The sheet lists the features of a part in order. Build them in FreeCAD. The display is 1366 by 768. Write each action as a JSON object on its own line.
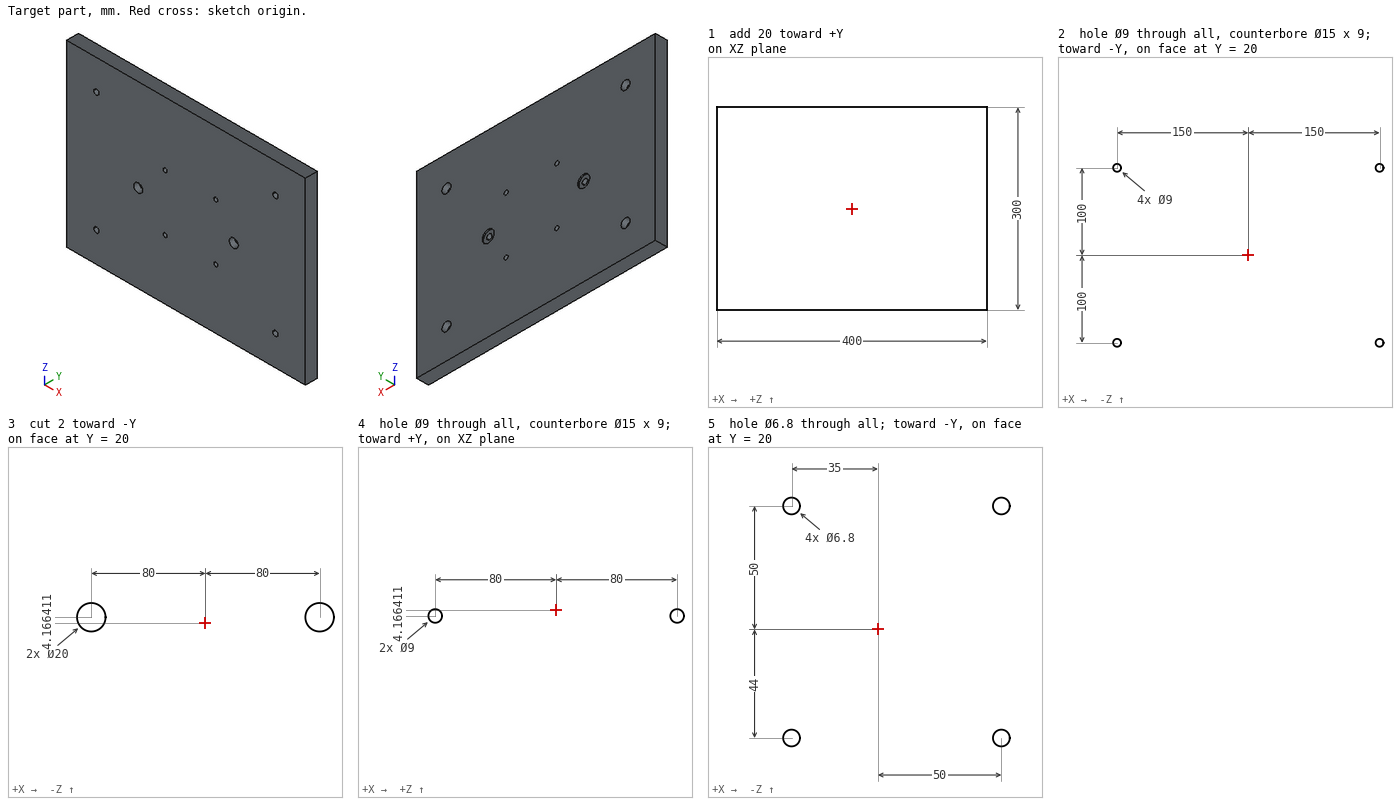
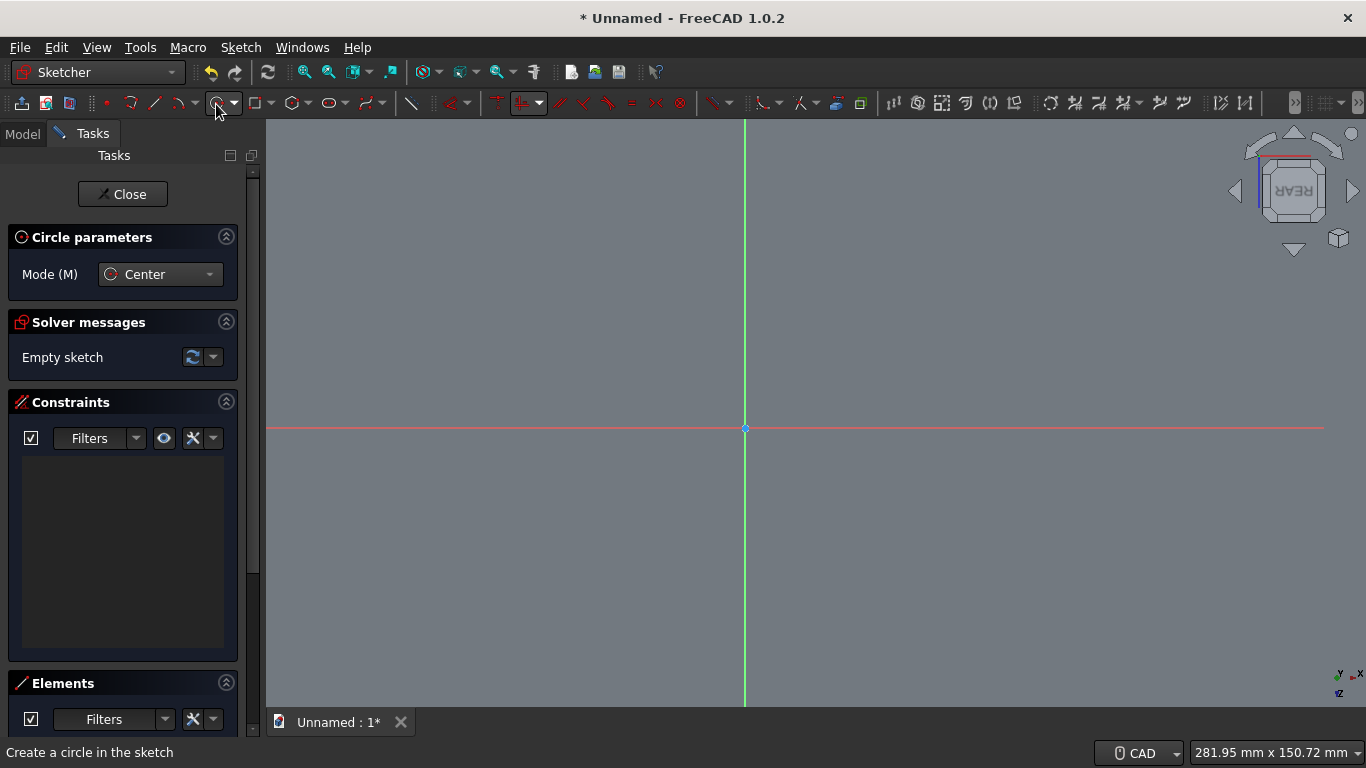
{"action": "left_click", "coordinate": [433, 412]}
{"action": "left_click", "coordinate": [461, 384]}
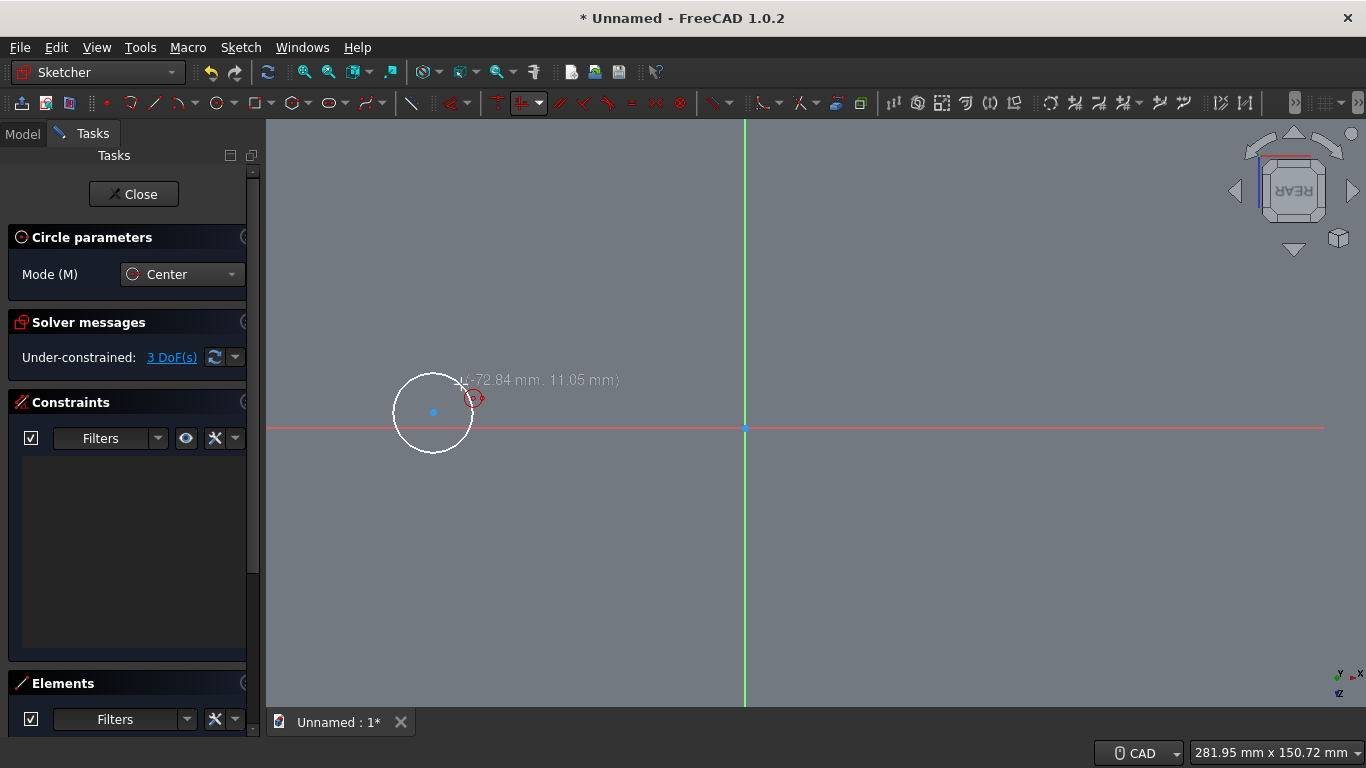
{"action": "left_click", "coordinate": [1057, 412]}
{"action": "left_click", "coordinate": [1085, 384]}
{"action": "key", "text": "Escape"}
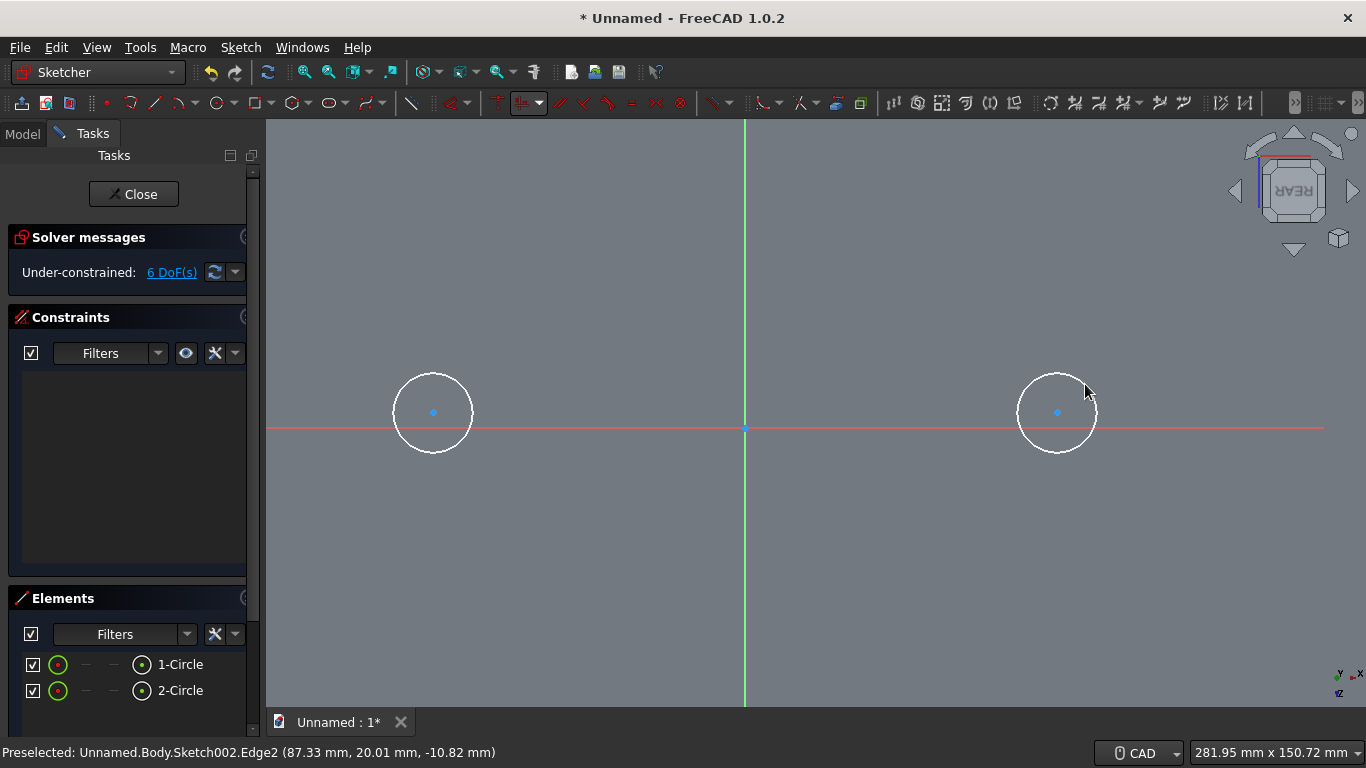
{"action": "left_click", "coordinate": [461, 385]}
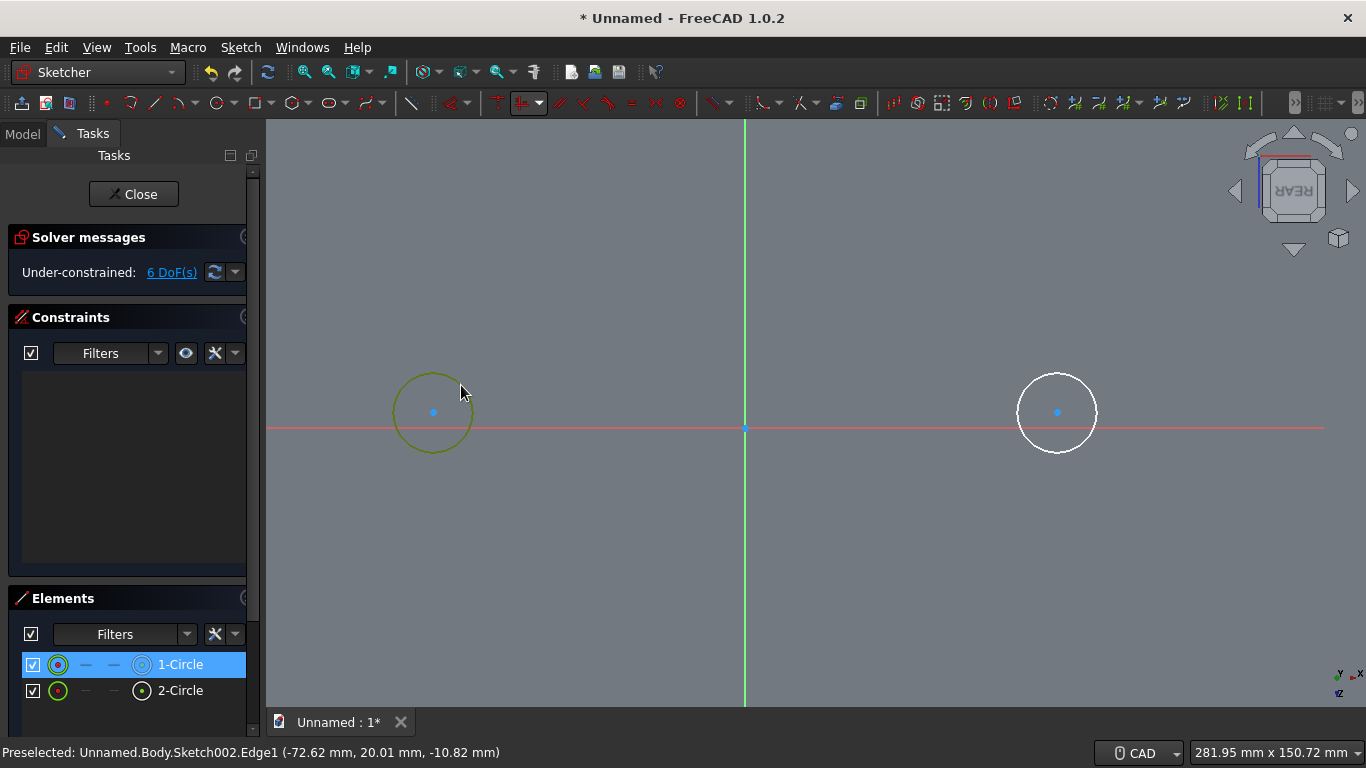
{"action": "left_click", "coordinate": [1085, 385]}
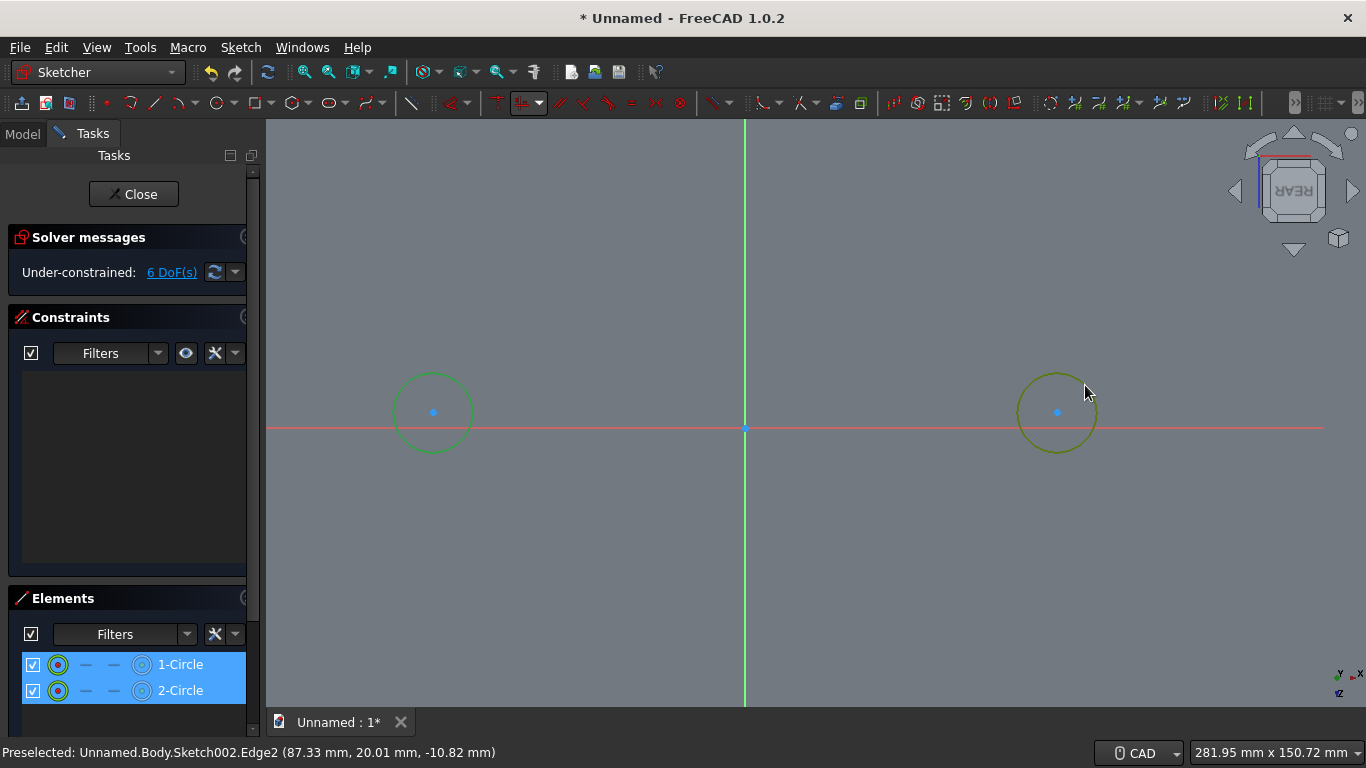
{"action": "left_click", "coordinate": [632, 104]}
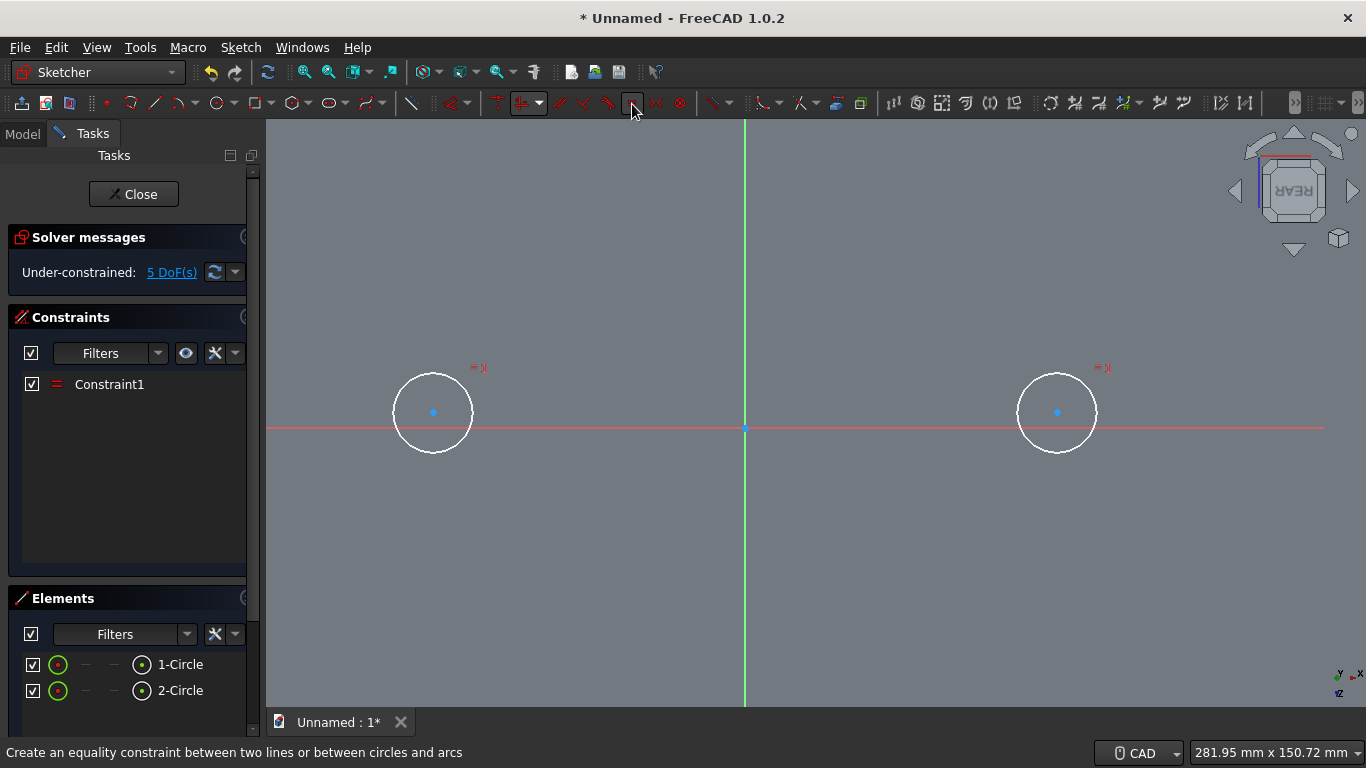
{"action": "left_click", "coordinate": [433, 413]}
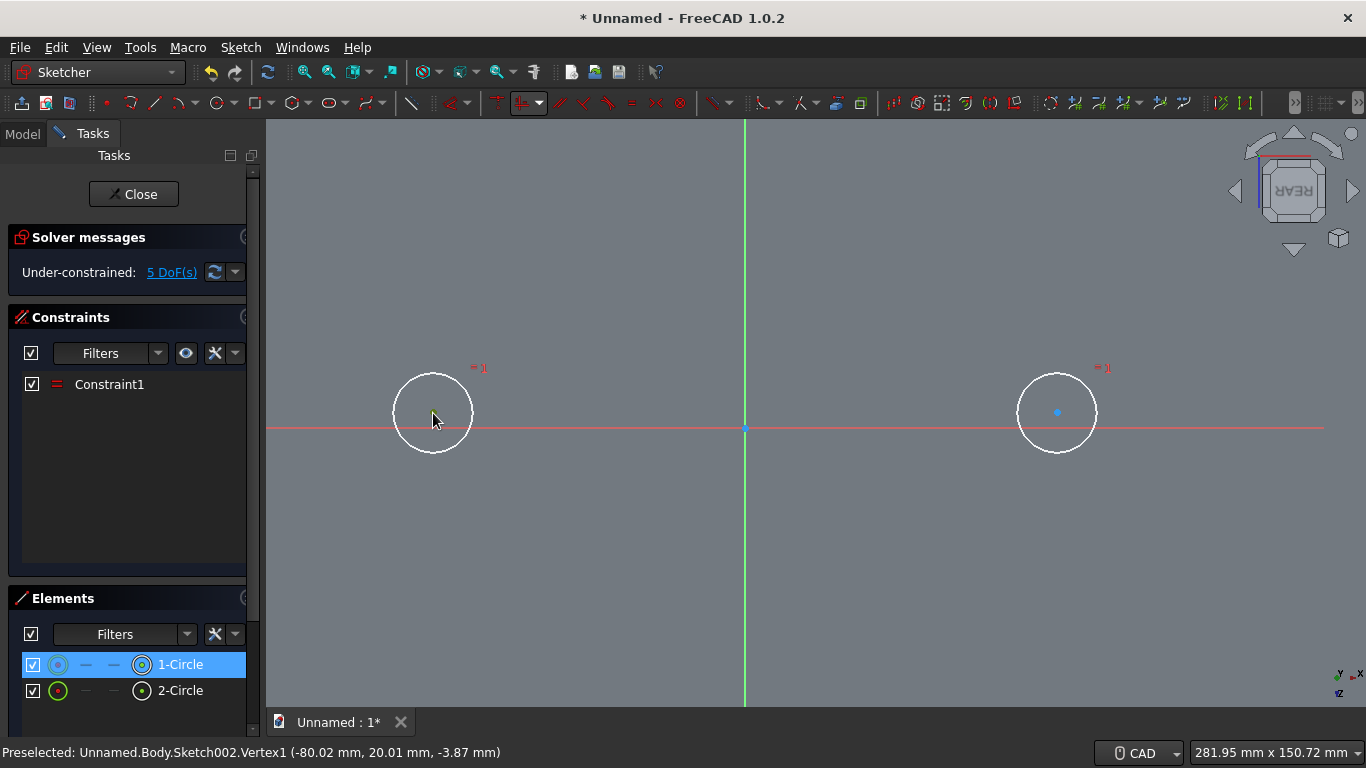
{"action": "left_click", "coordinate": [1057, 413]}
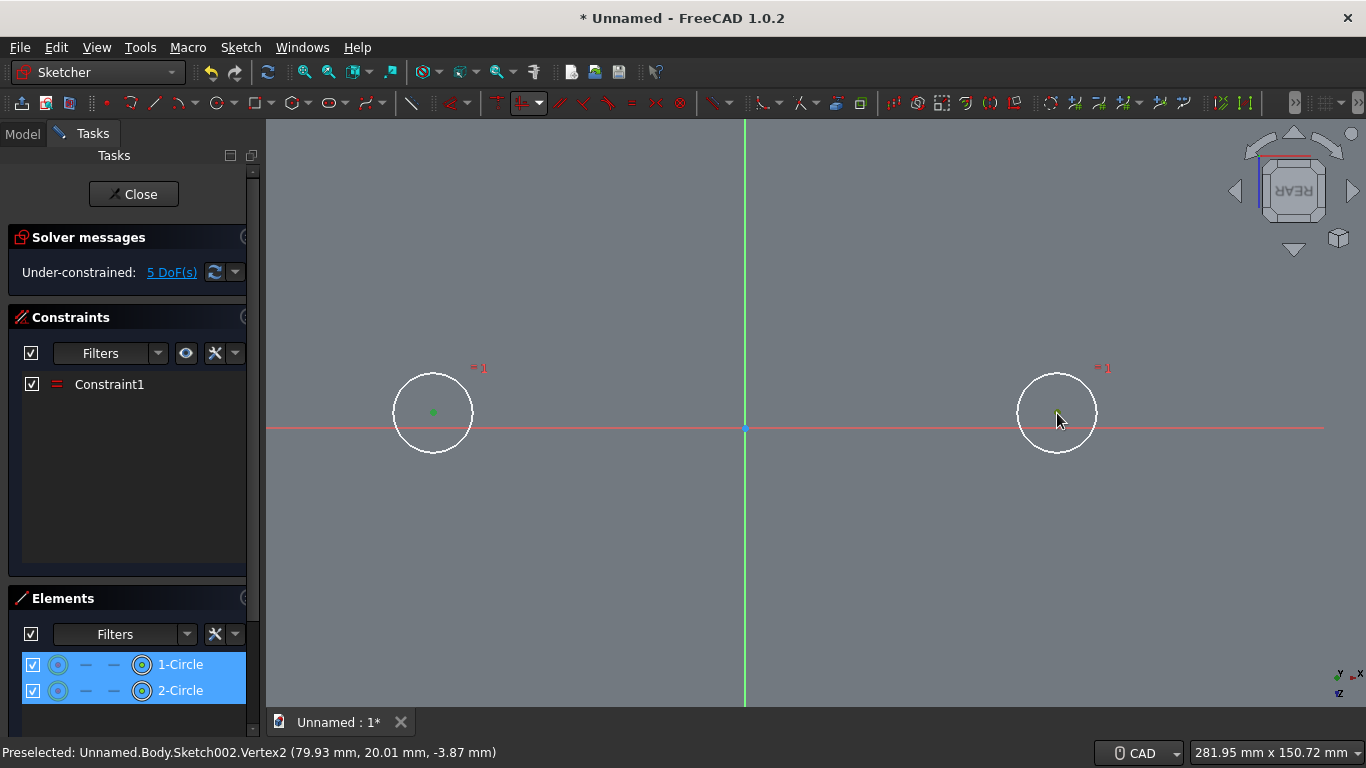
{"action": "key", "text": "h"}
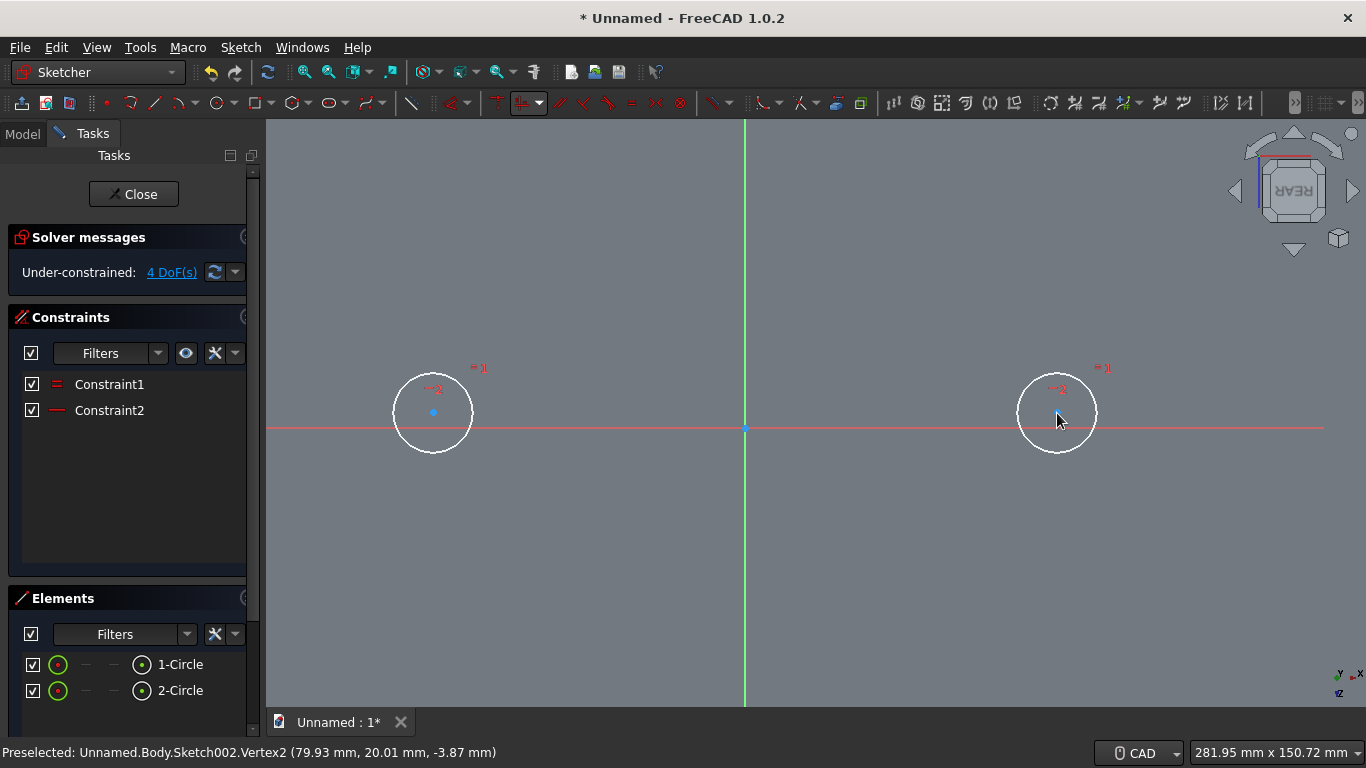
{"action": "left_click", "coordinate": [450, 104]}